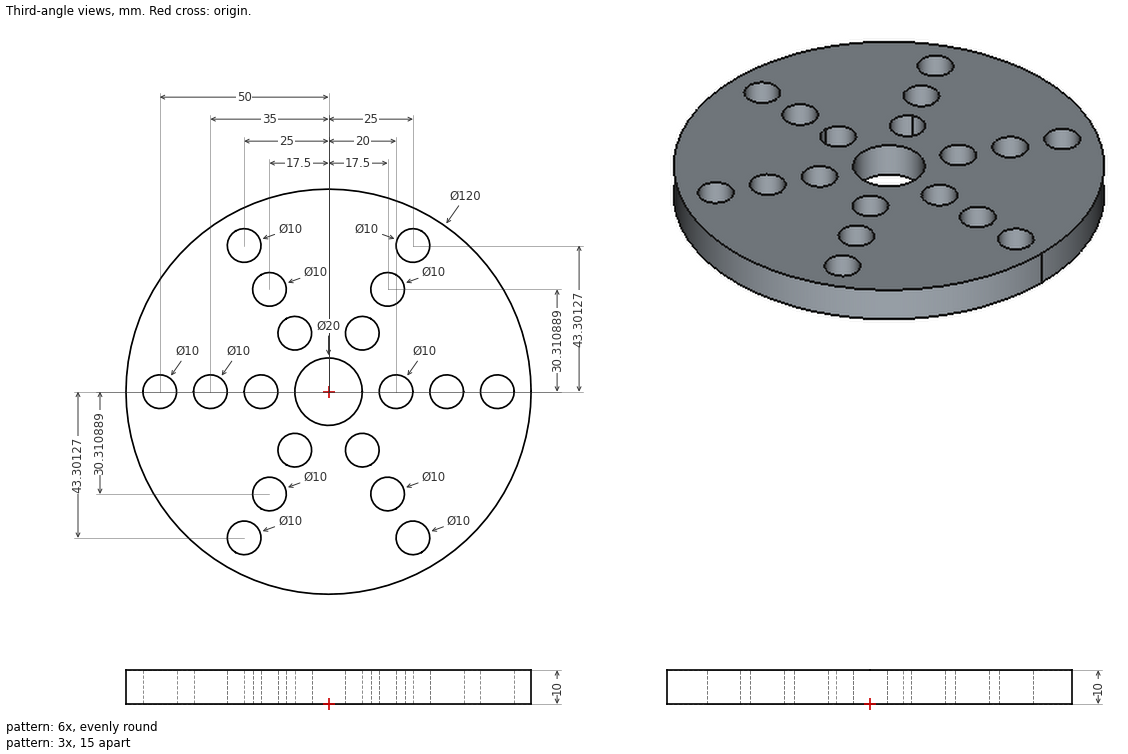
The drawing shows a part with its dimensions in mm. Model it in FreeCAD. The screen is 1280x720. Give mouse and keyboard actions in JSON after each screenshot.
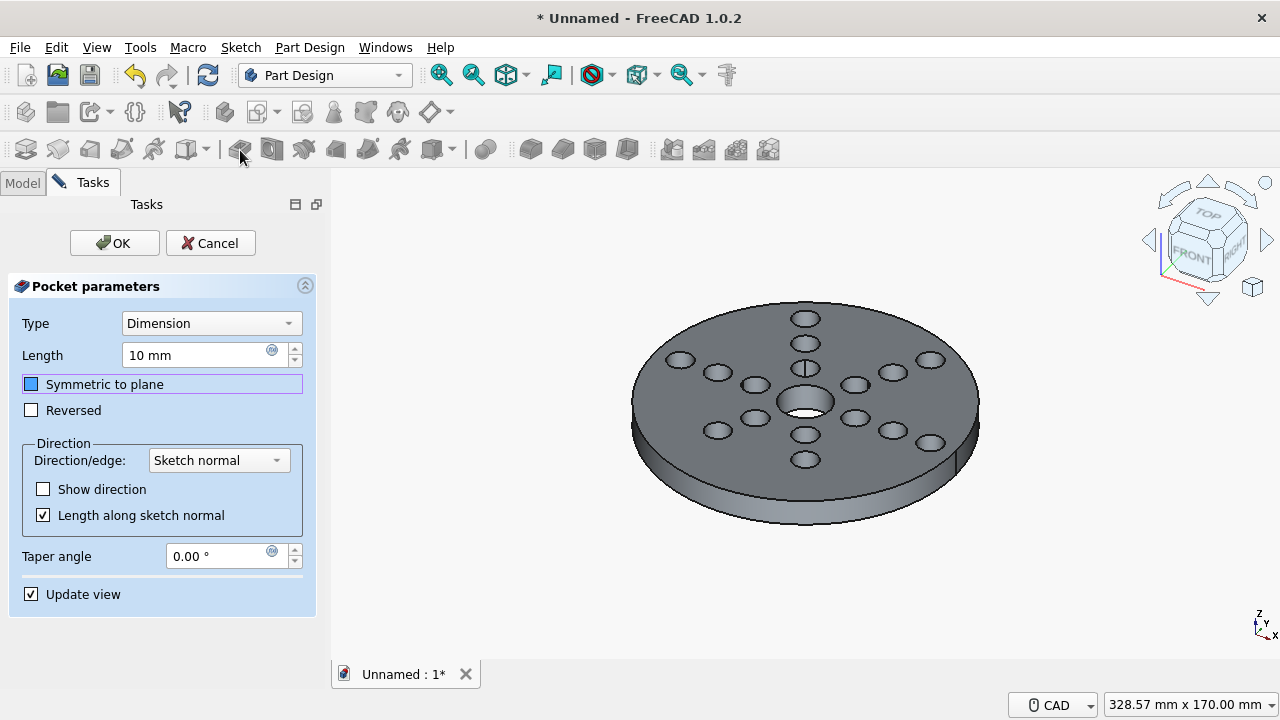
{"action": "left_click", "coordinate": [115, 243]}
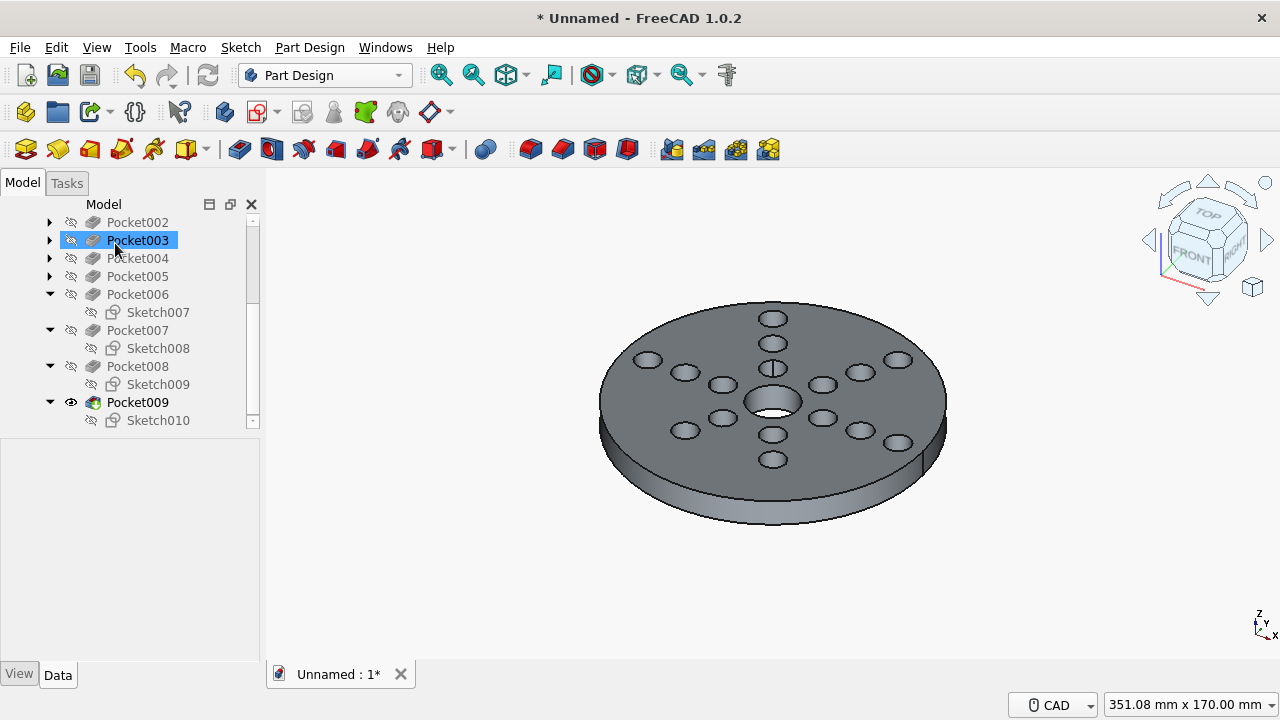
{"action": "left_click", "coordinate": [823, 351]}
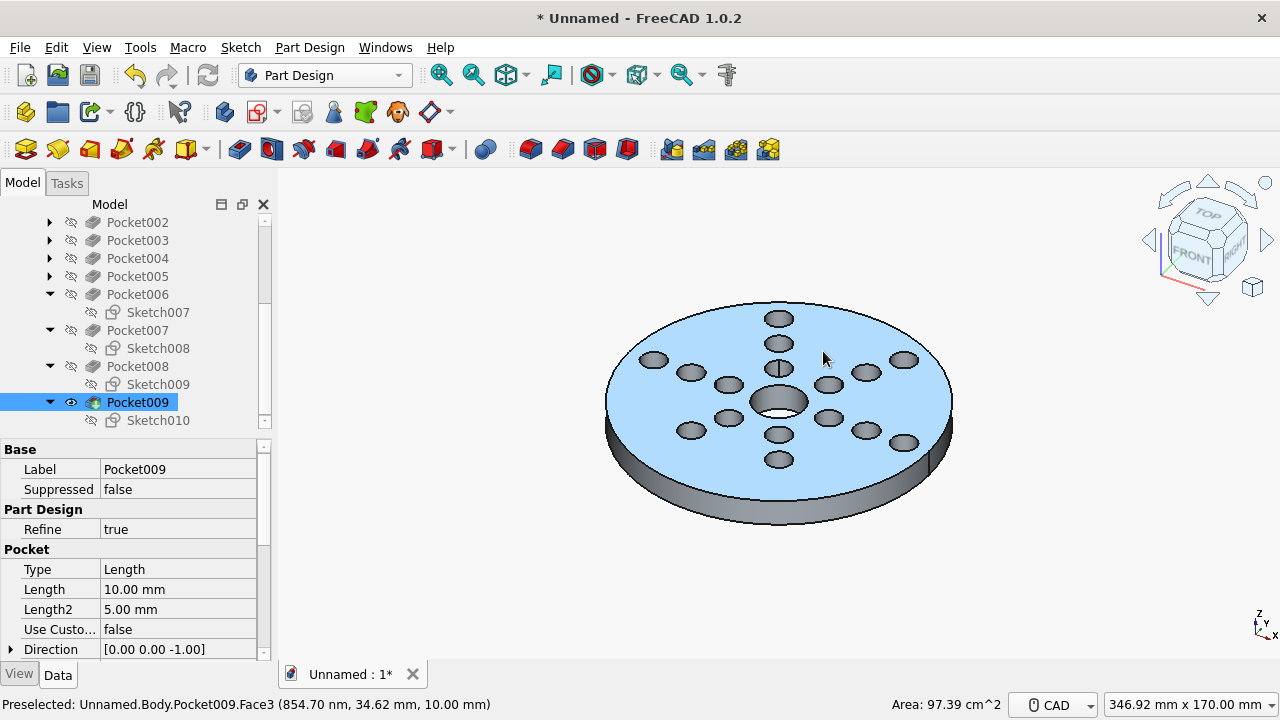
{"action": "left_click", "coordinate": [258, 112]}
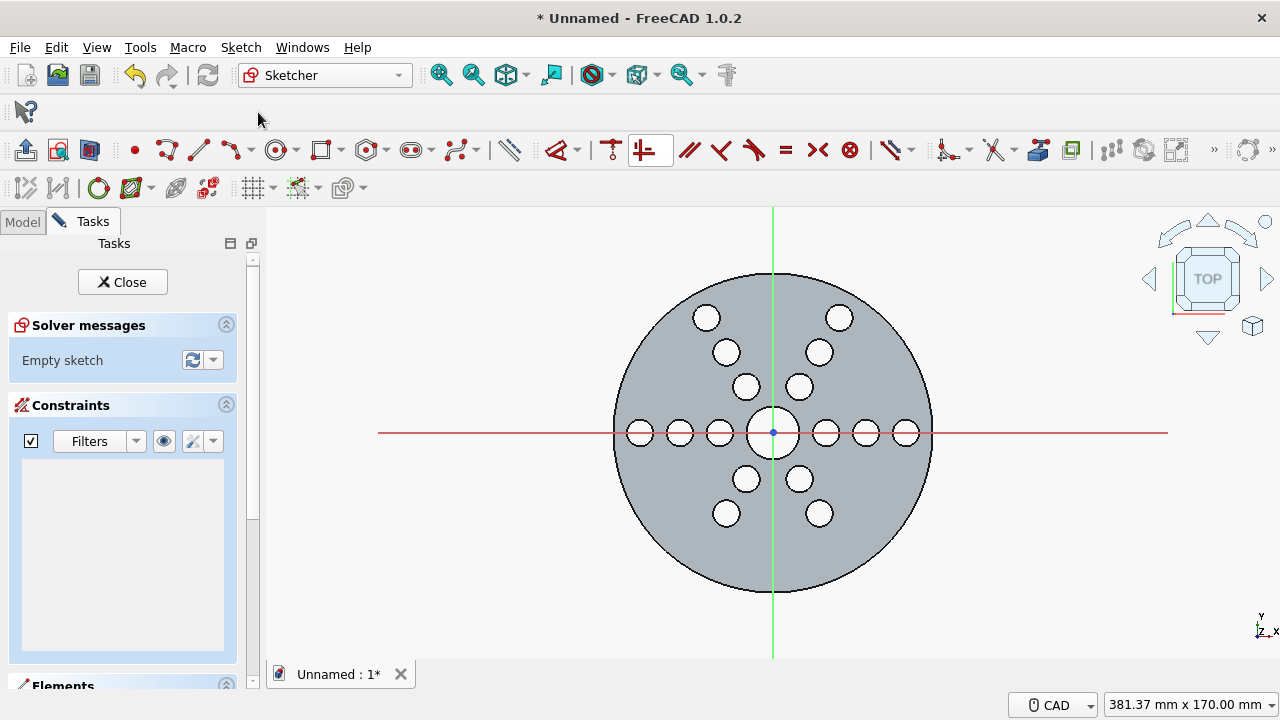
{"action": "scroll", "coordinate": [707, 560], "scroll_direction": "up", "scroll_amount": 12}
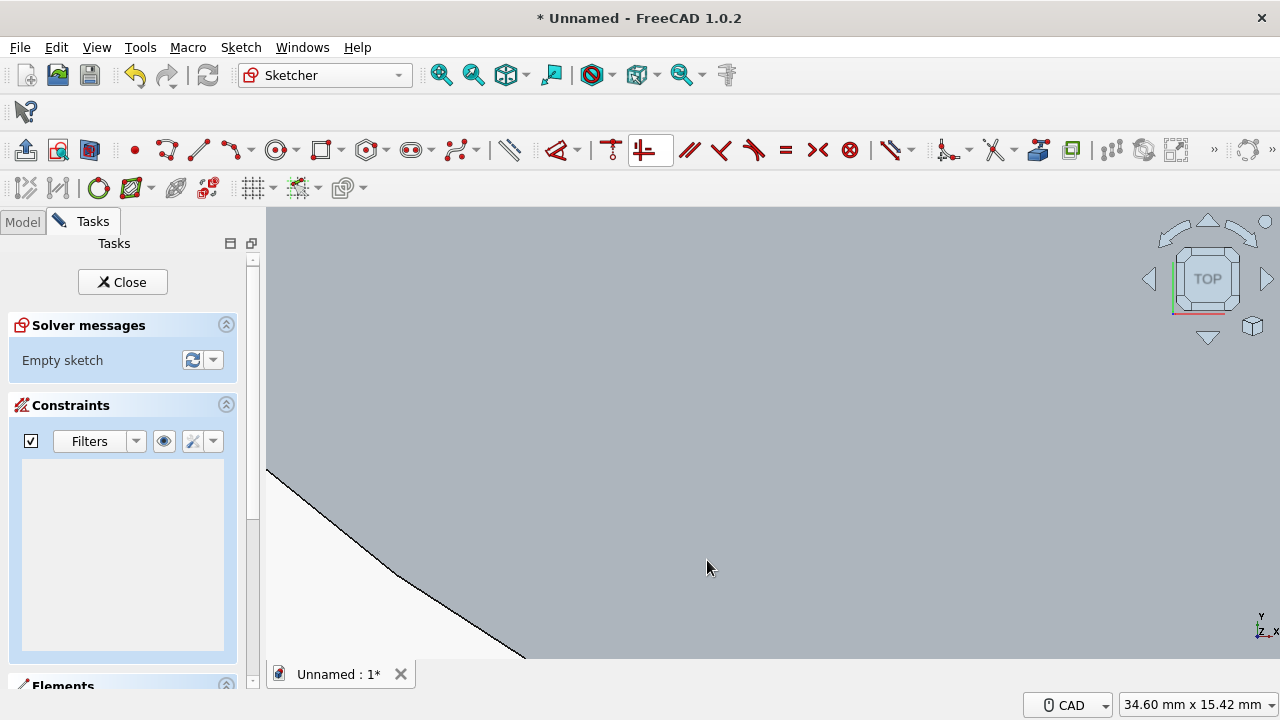
{"action": "left_click", "coordinate": [276, 150]}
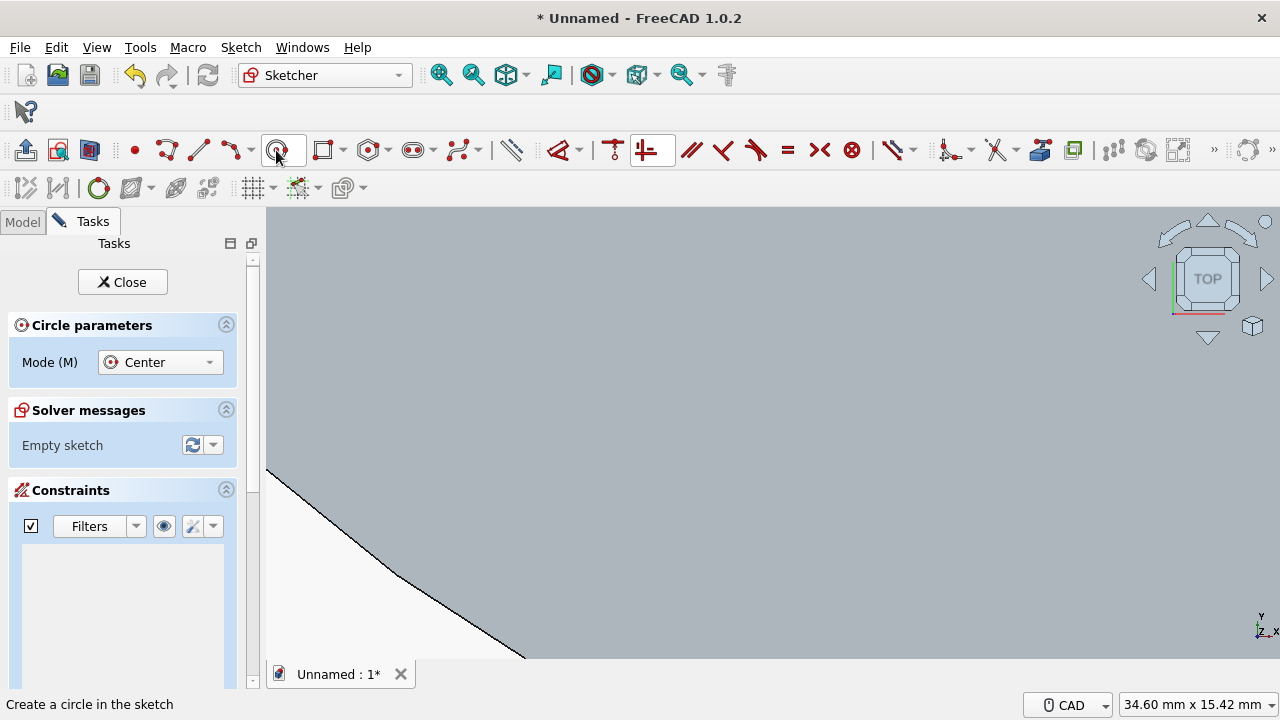
{"action": "left_click", "coordinate": [697, 421]}
{"action": "left_click", "coordinate": [801, 318]}
{"action": "key", "text": "Escape"}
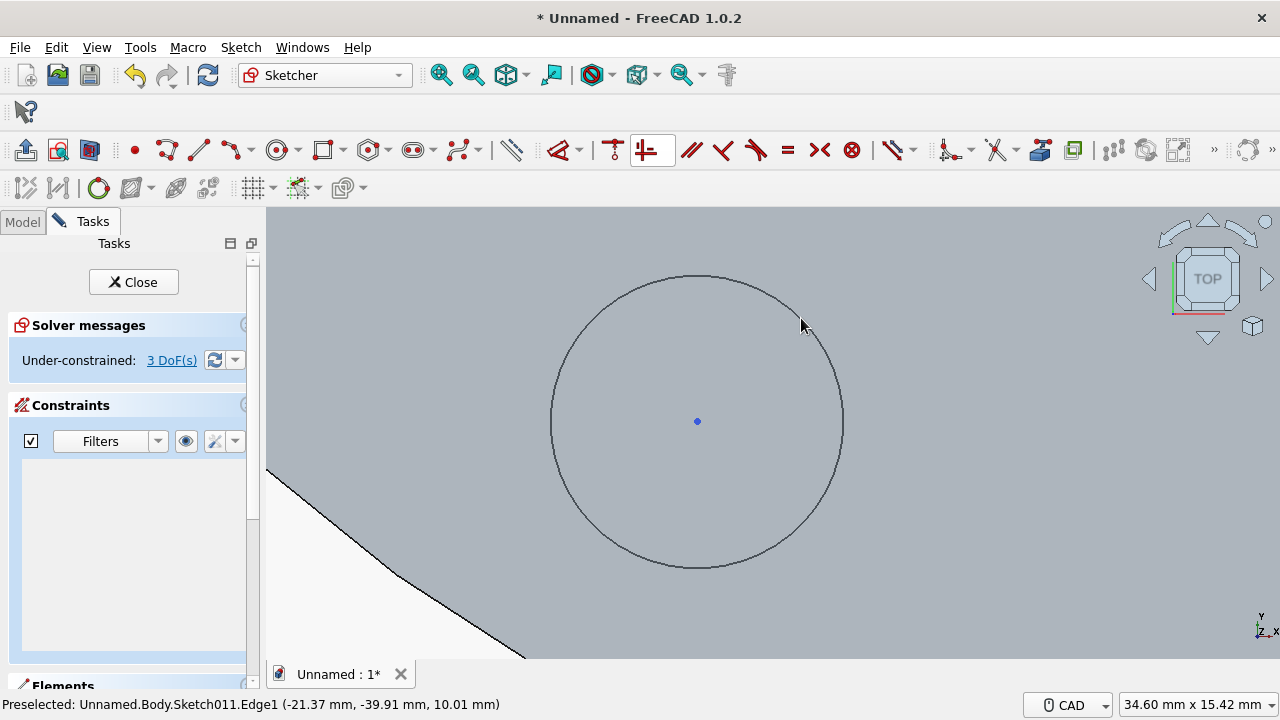
{"action": "left_click", "coordinate": [558, 150]}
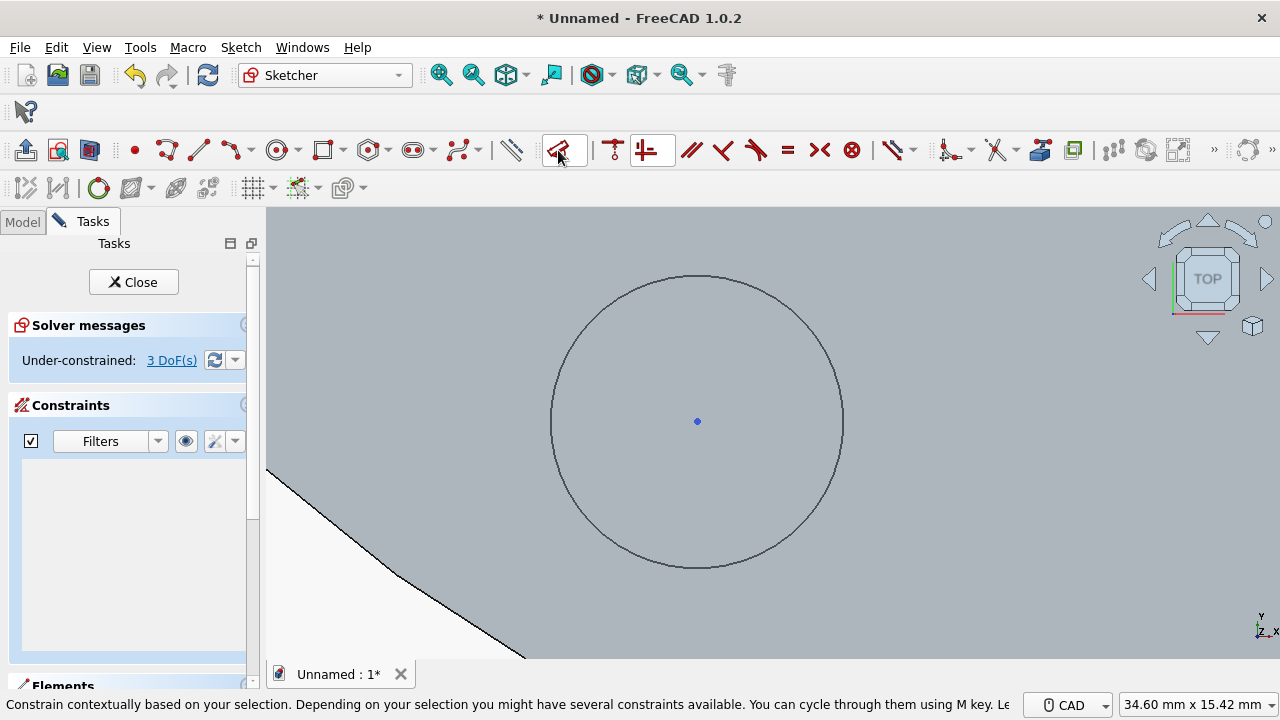
{"action": "left_click", "coordinate": [800, 318]}
{"action": "left_click", "coordinate": [823, 295]}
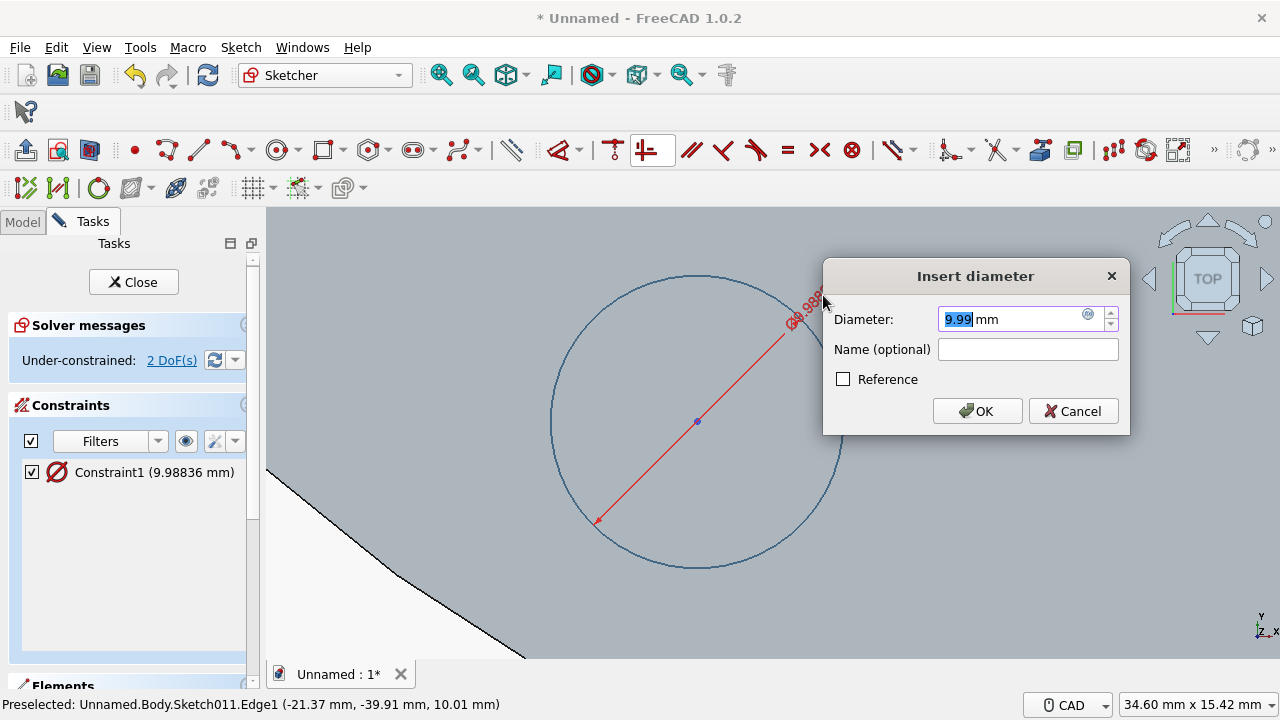
{"action": "type", "text": "10"}
{"action": "key", "text": "Return"}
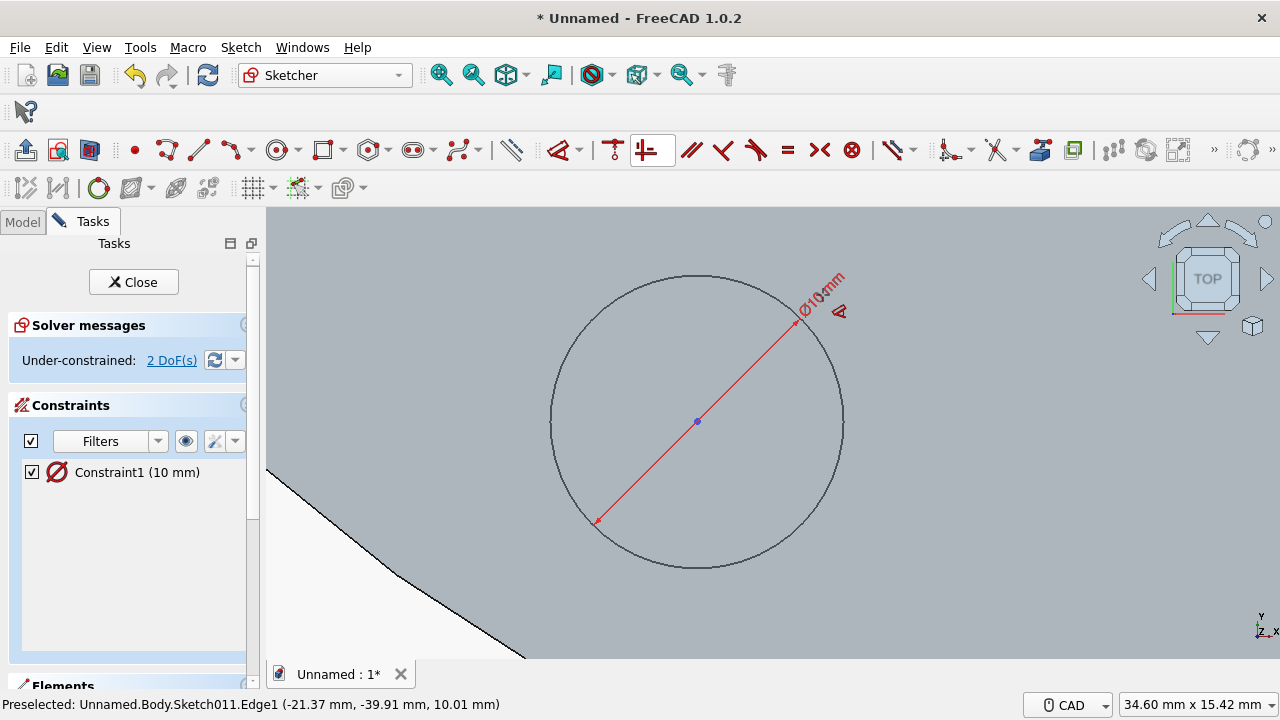
{"action": "left_click", "coordinate": [697, 422]}
{"action": "left_click", "coordinate": [906, 456]}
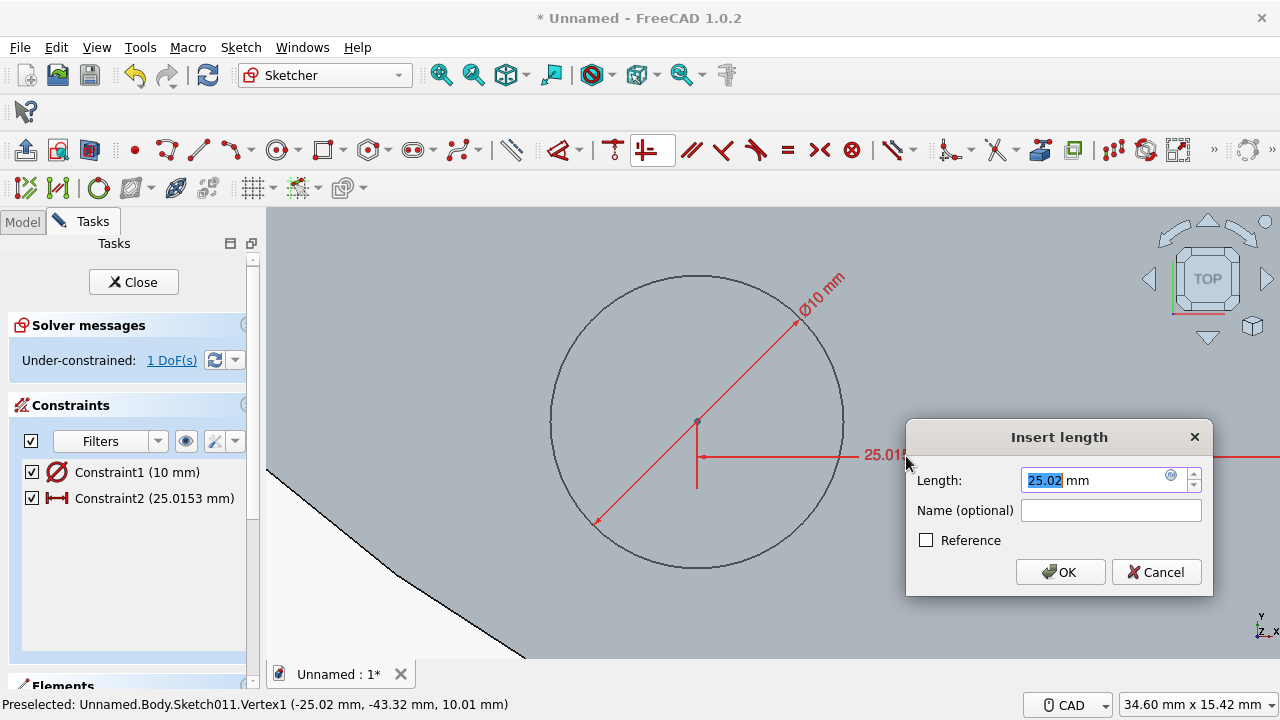
{"action": "type", "text": "25"}
{"action": "key", "text": "Return"}